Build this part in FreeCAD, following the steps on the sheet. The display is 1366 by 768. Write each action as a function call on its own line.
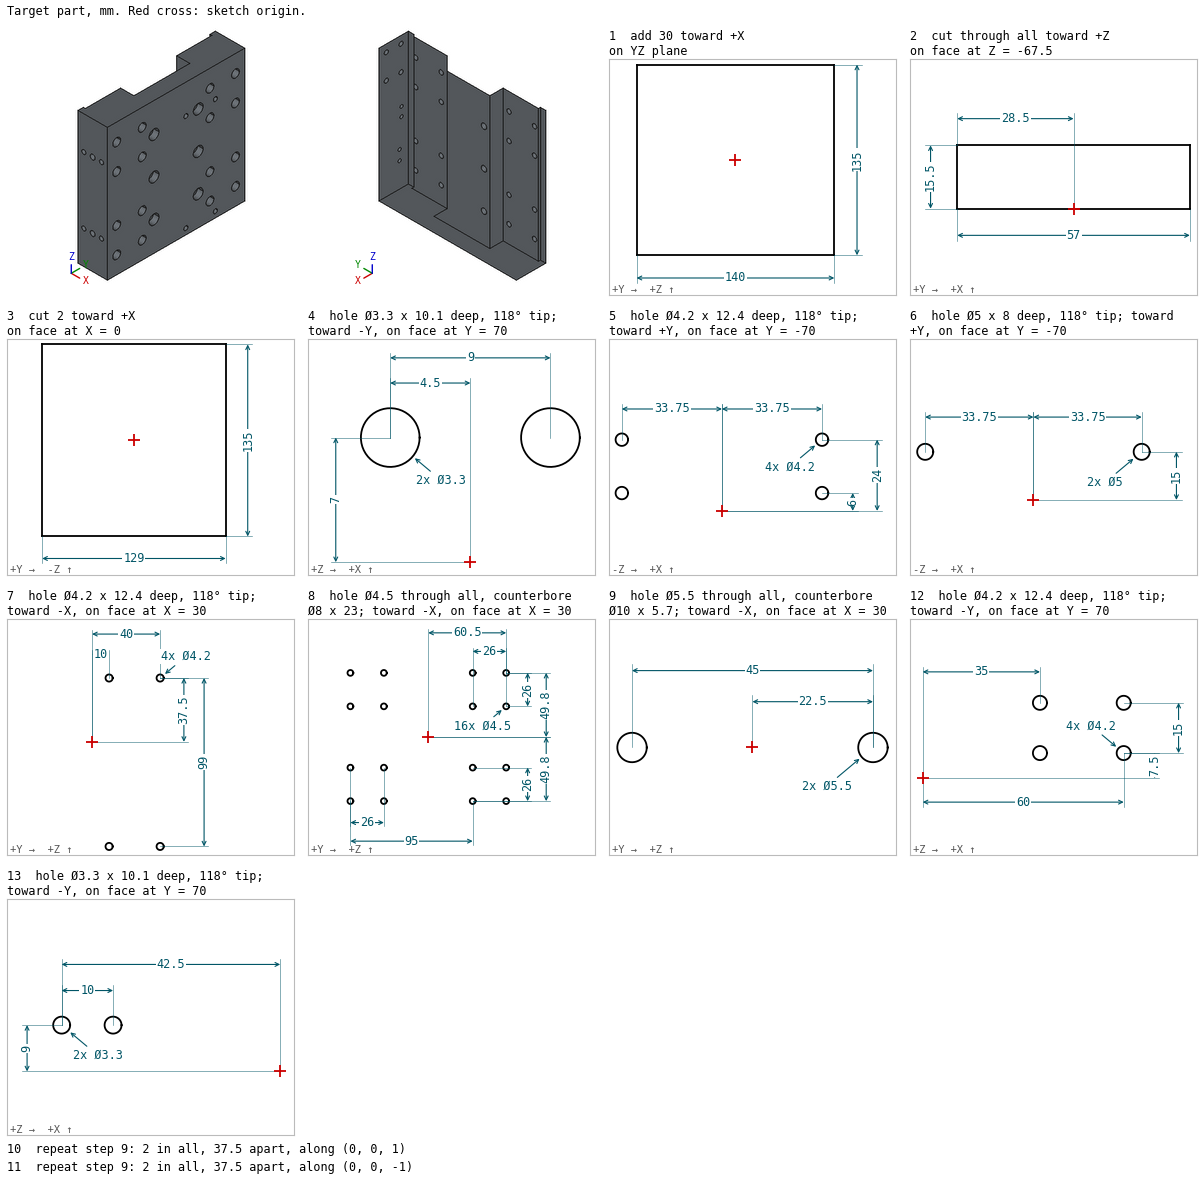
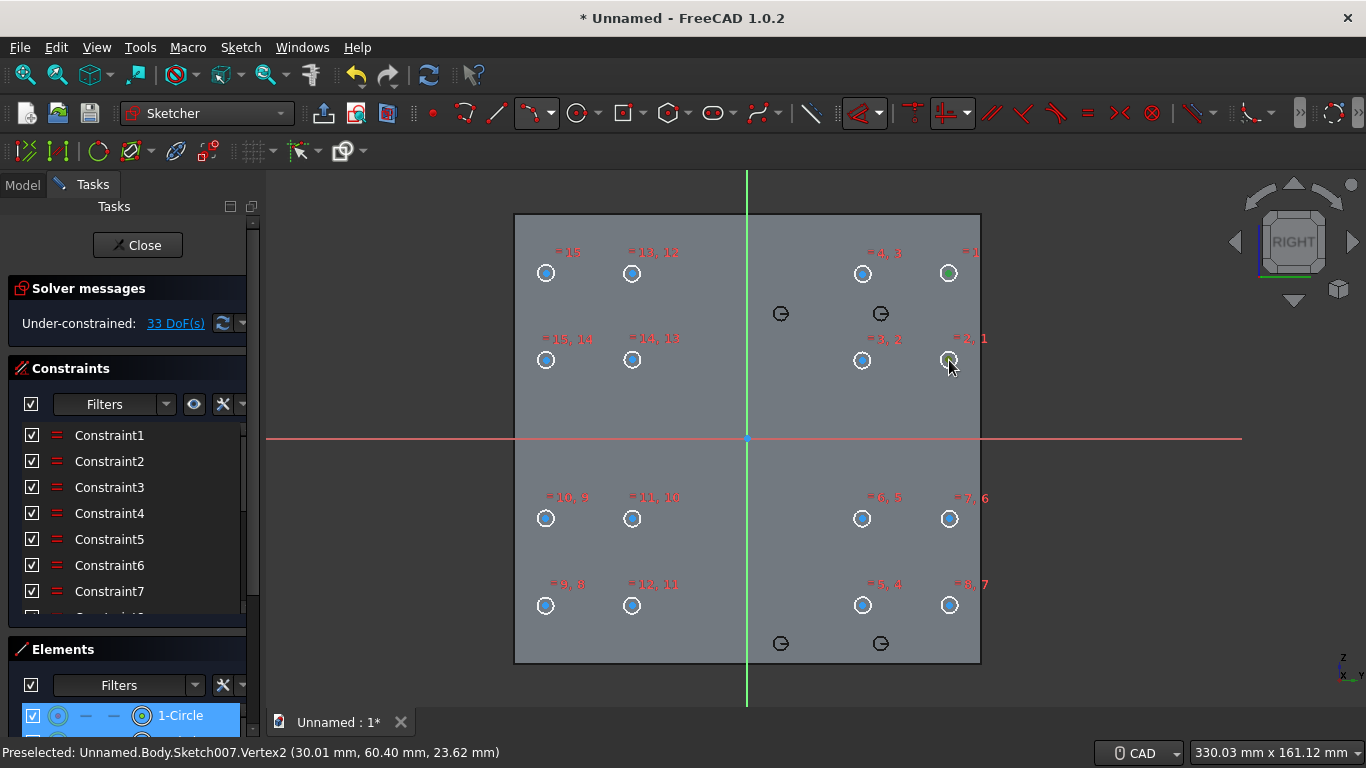
key(v)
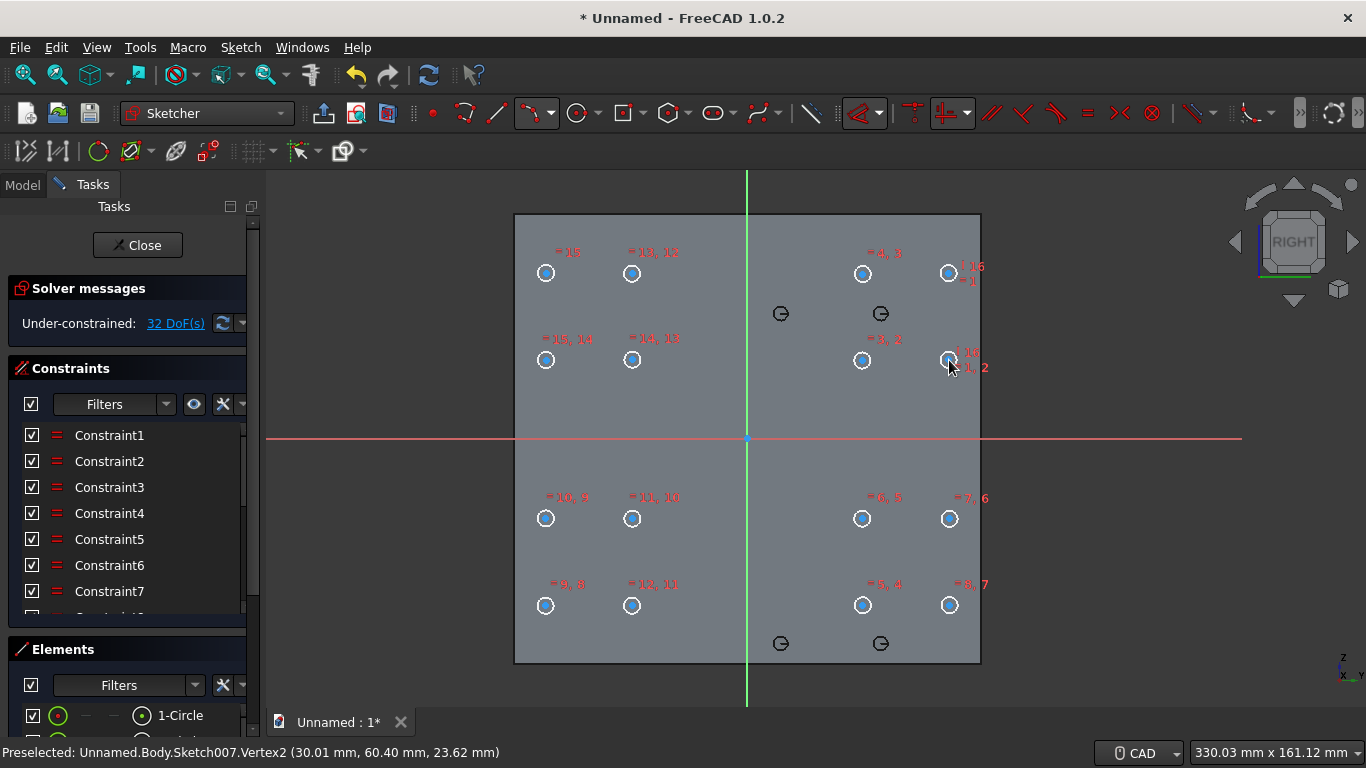
click(949, 360)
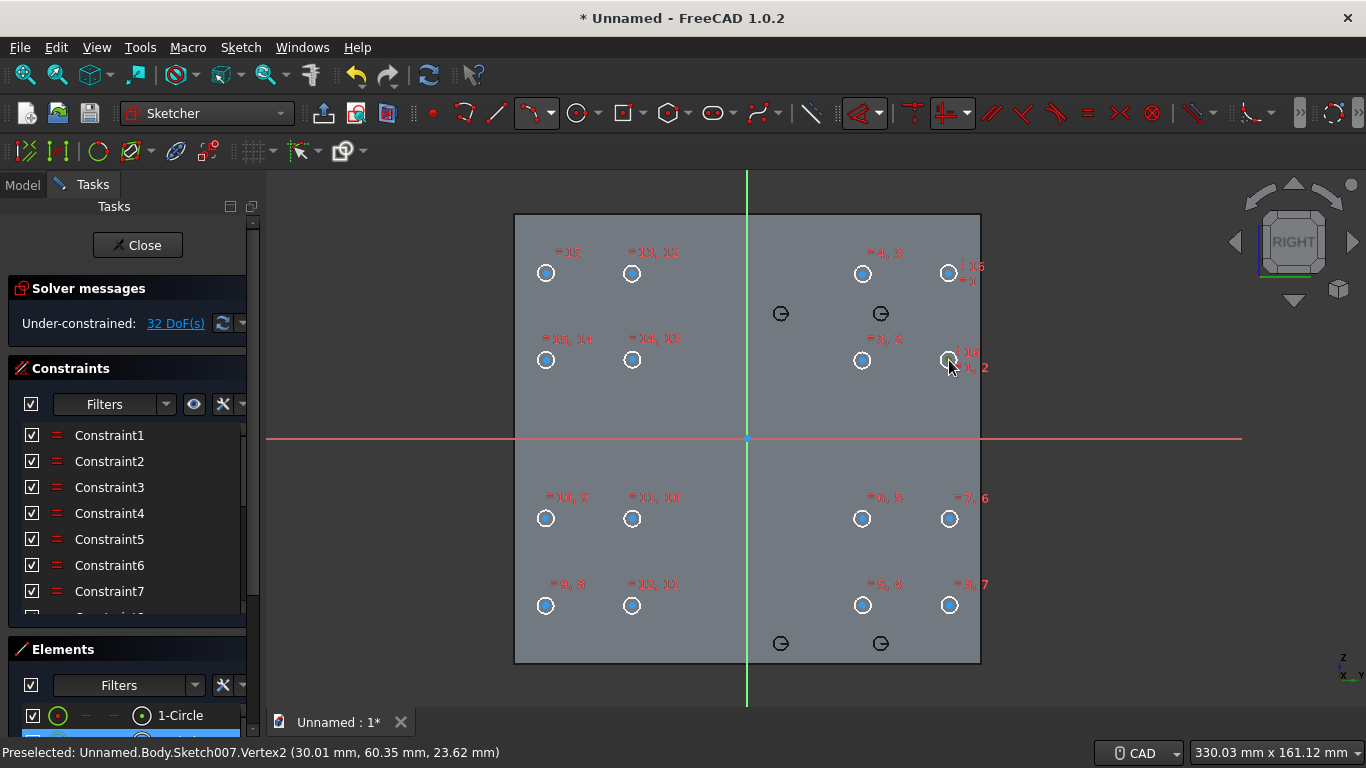
click(862, 360)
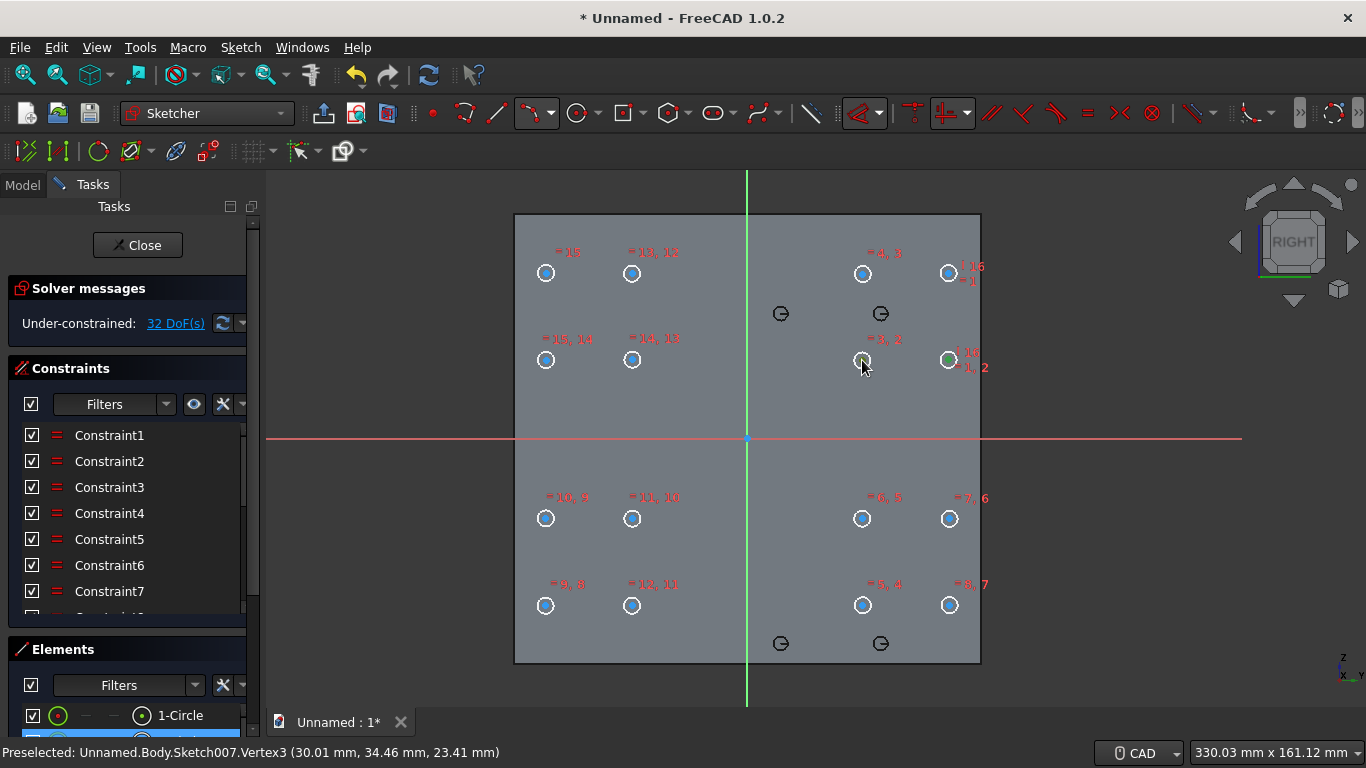
click(970, 114)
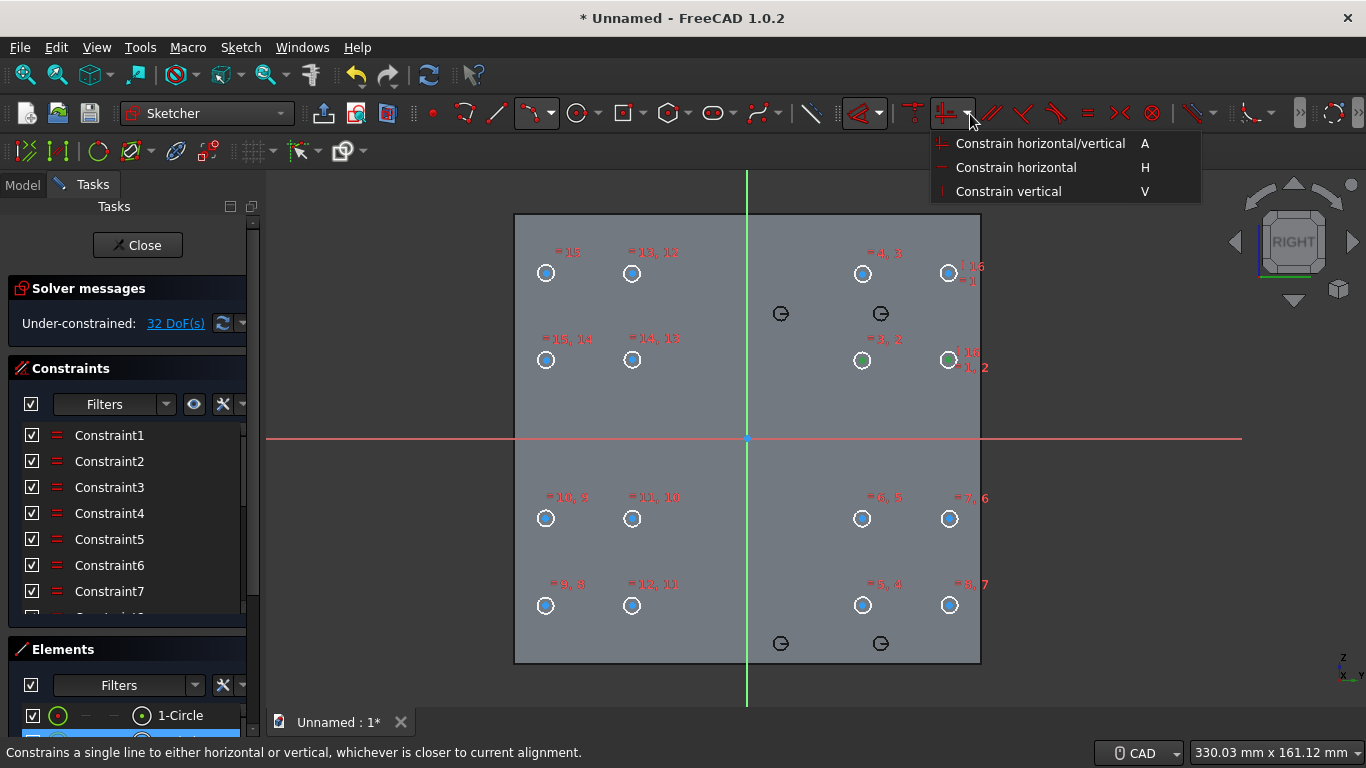
click(1066, 167)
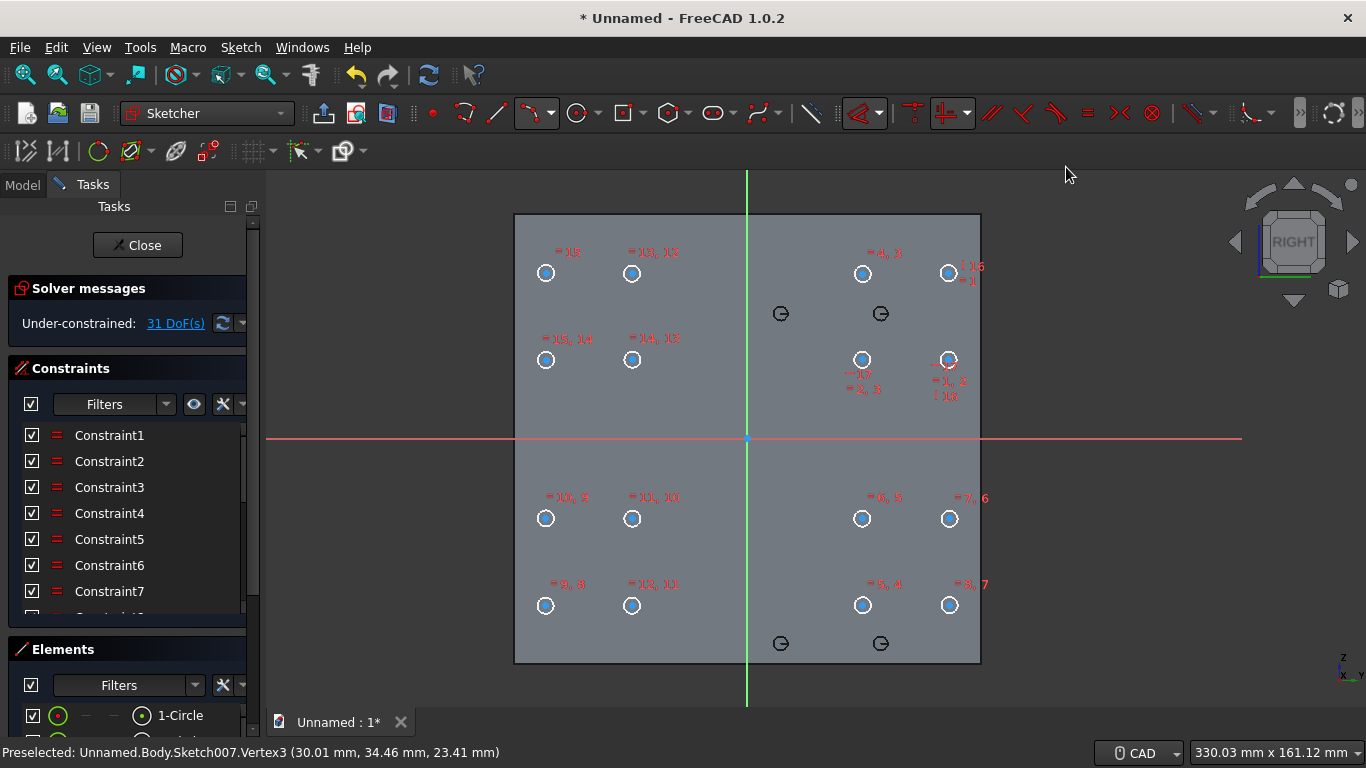
click(862, 360)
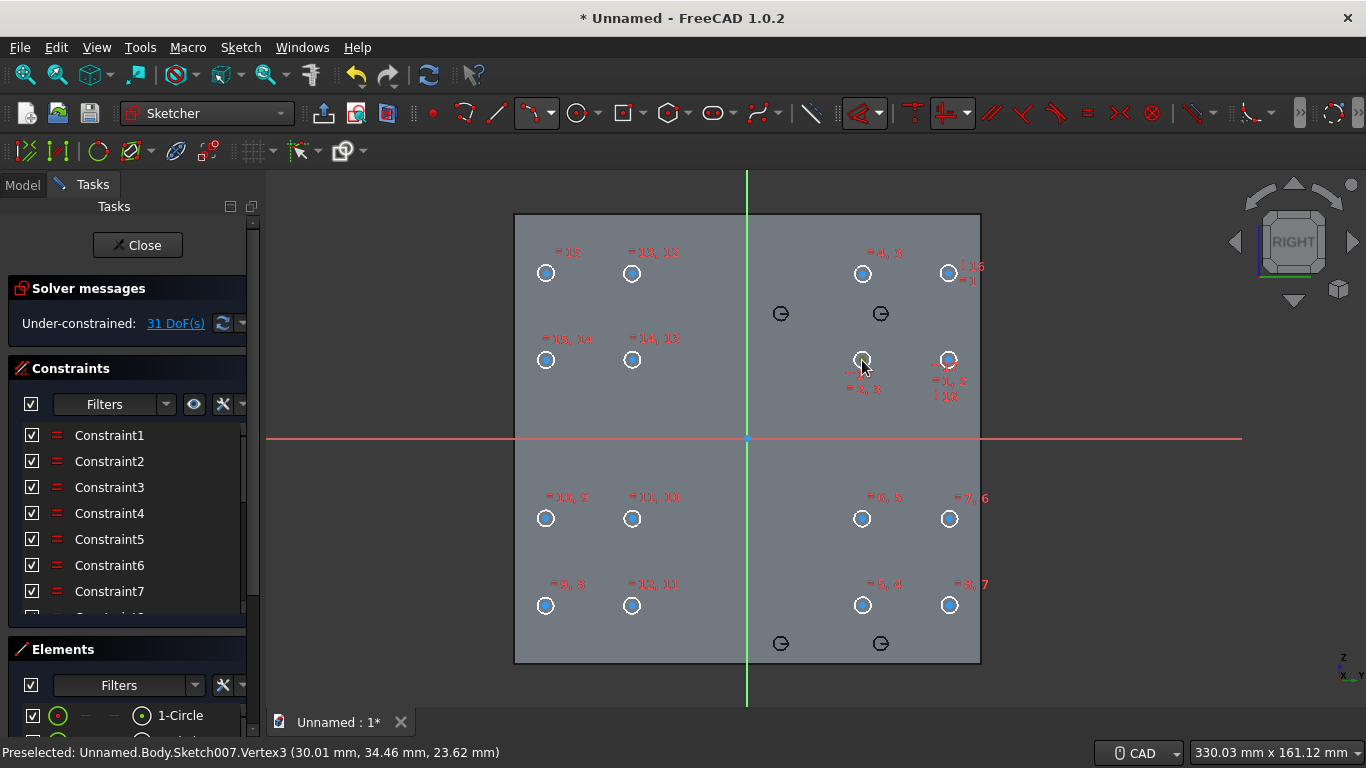
click(863, 274)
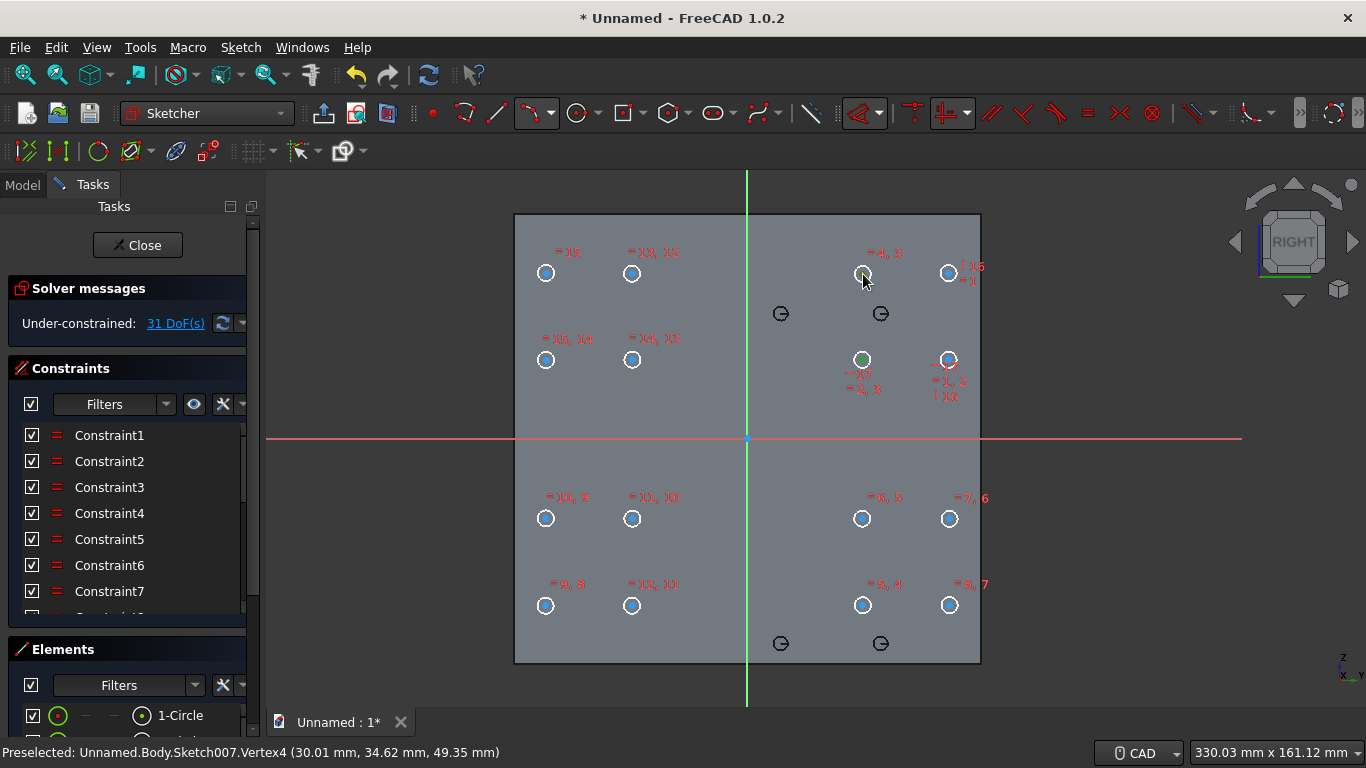
click(970, 114)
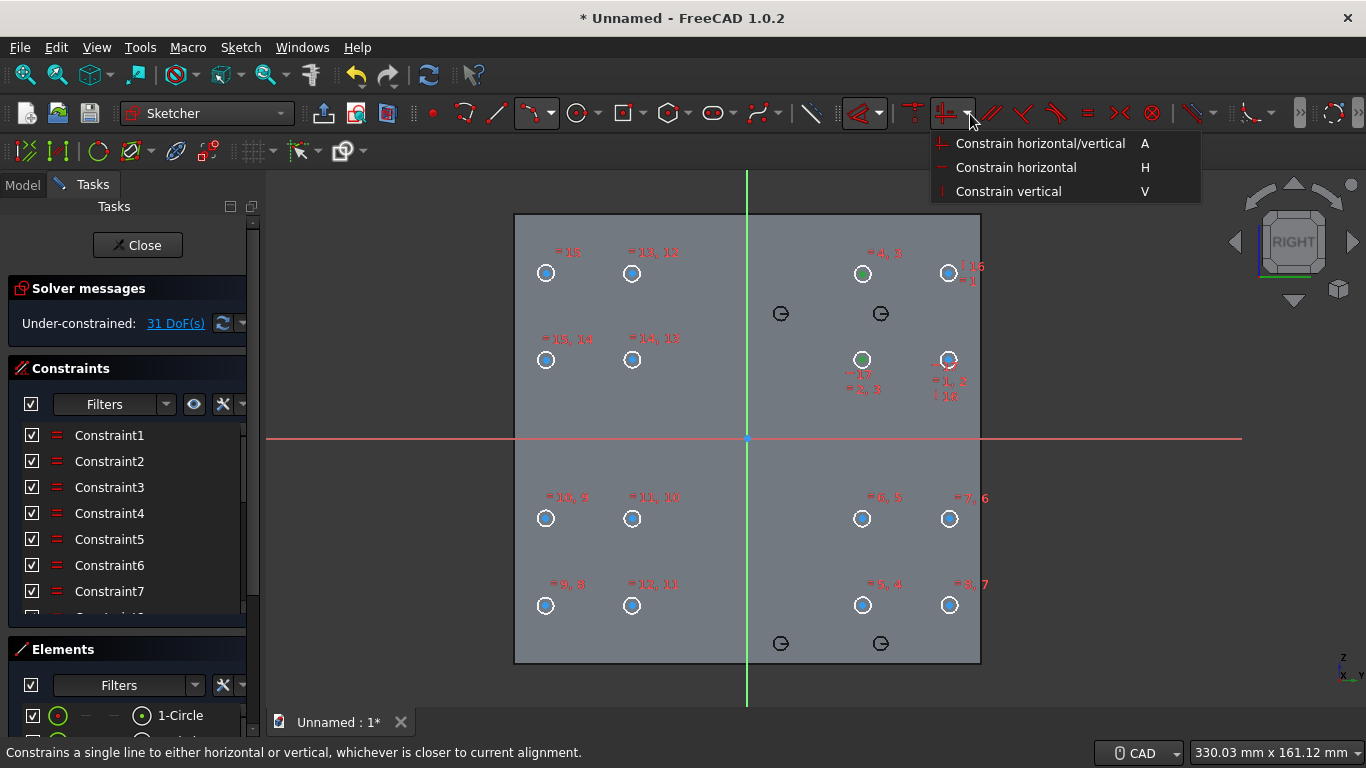
click(1066, 191)